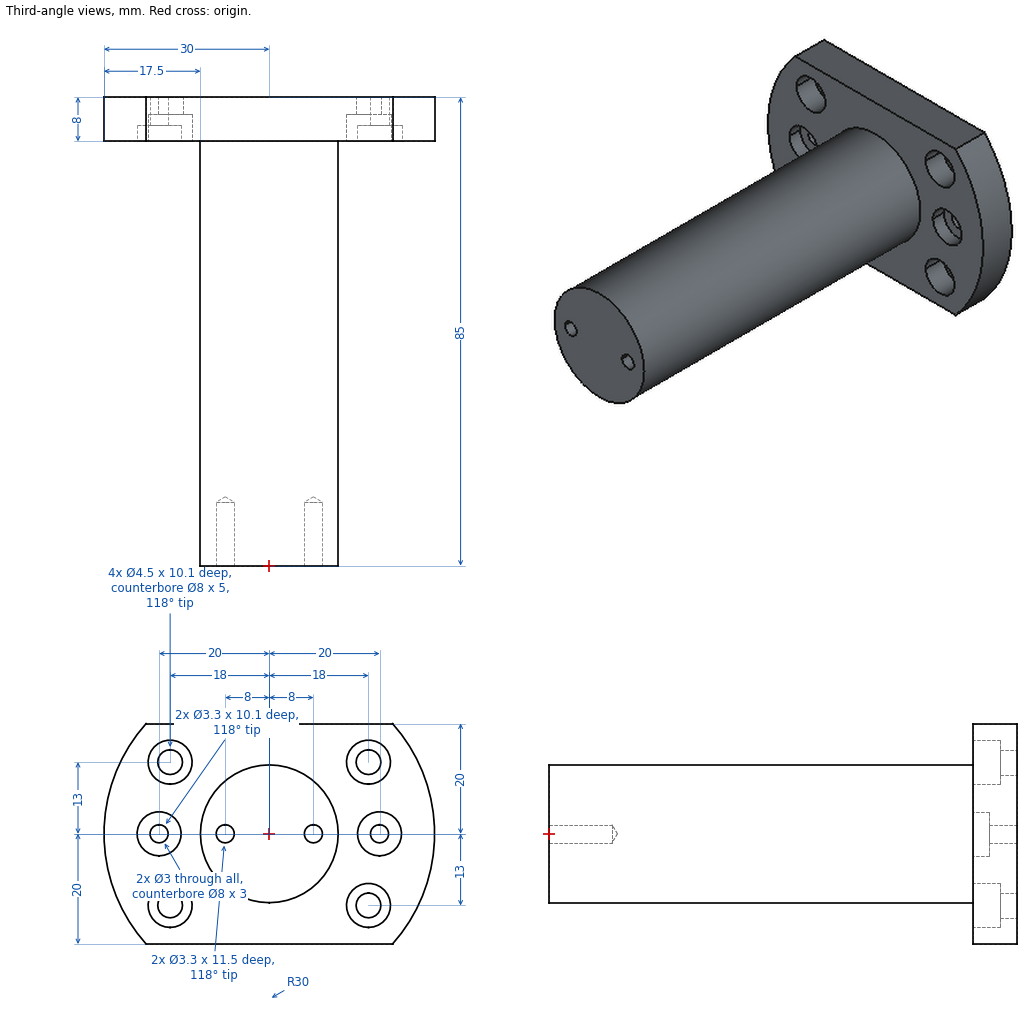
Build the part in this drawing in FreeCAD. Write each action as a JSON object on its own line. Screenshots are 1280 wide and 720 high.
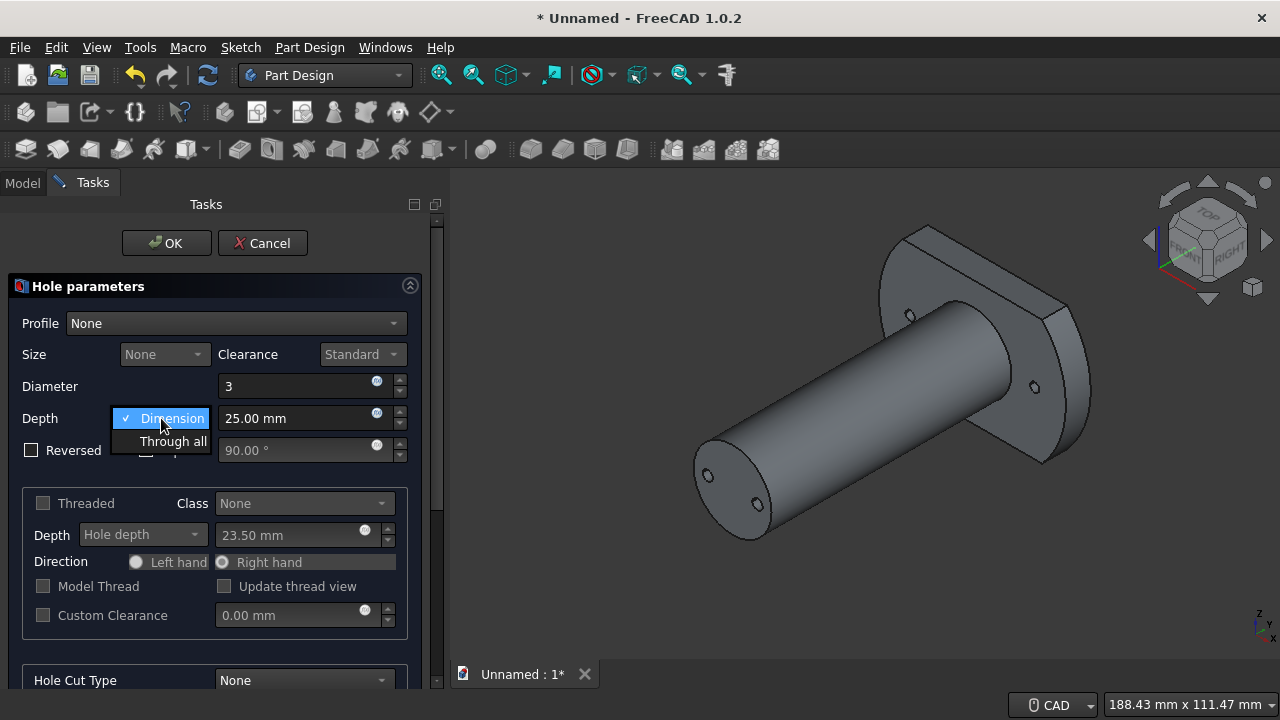
{"action": "left_click", "coordinate": [160, 442]}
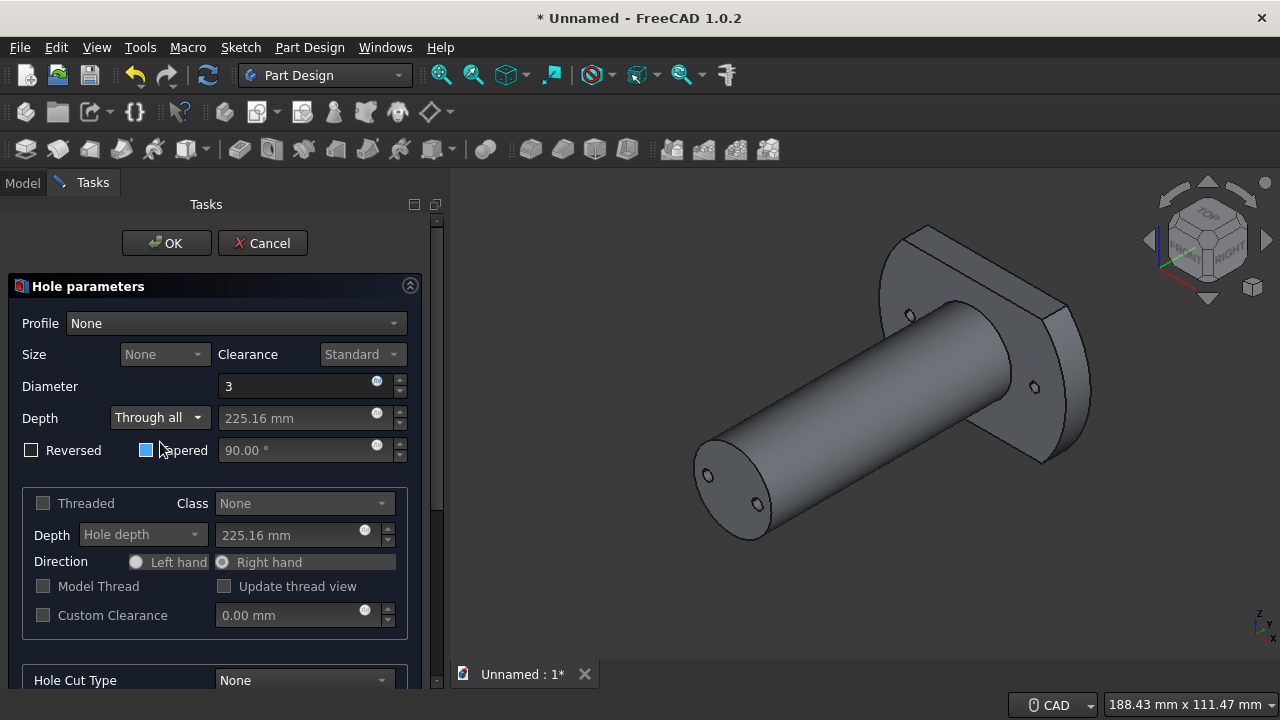
{"action": "scroll", "coordinate": [437, 451], "scroll_direction": "down", "scroll_amount": 2}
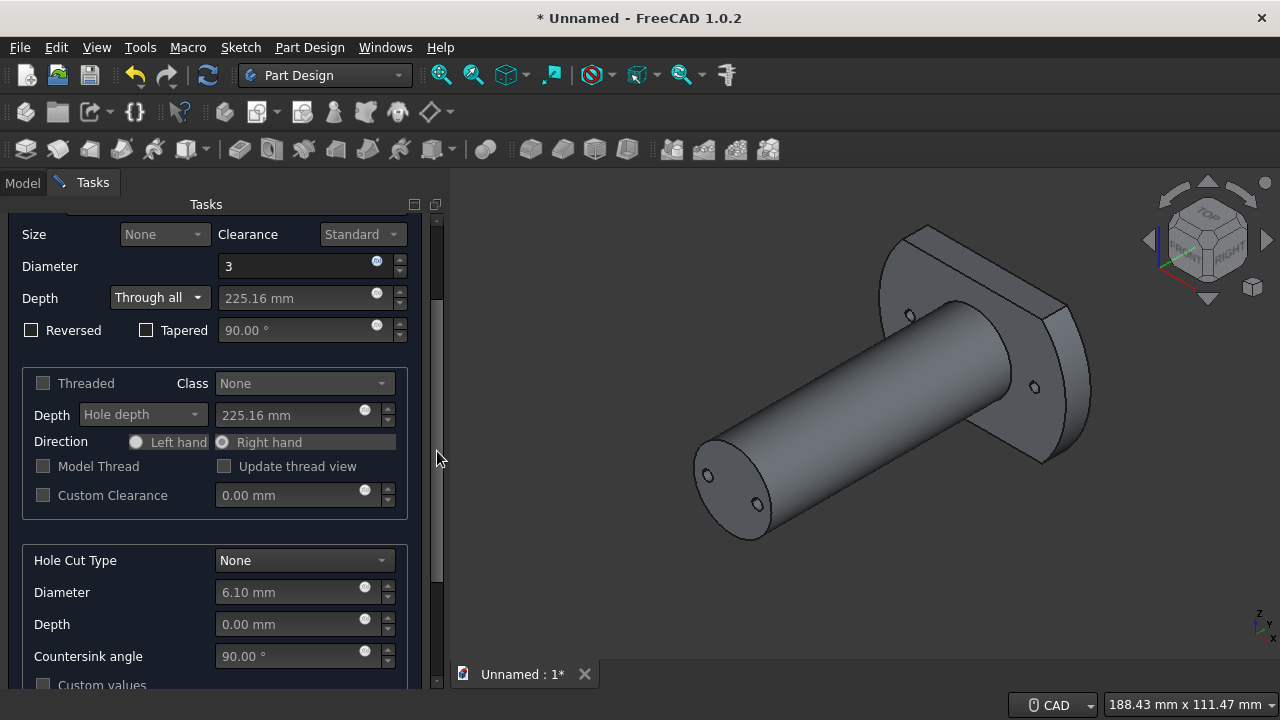
{"action": "left_click", "coordinate": [306, 560]}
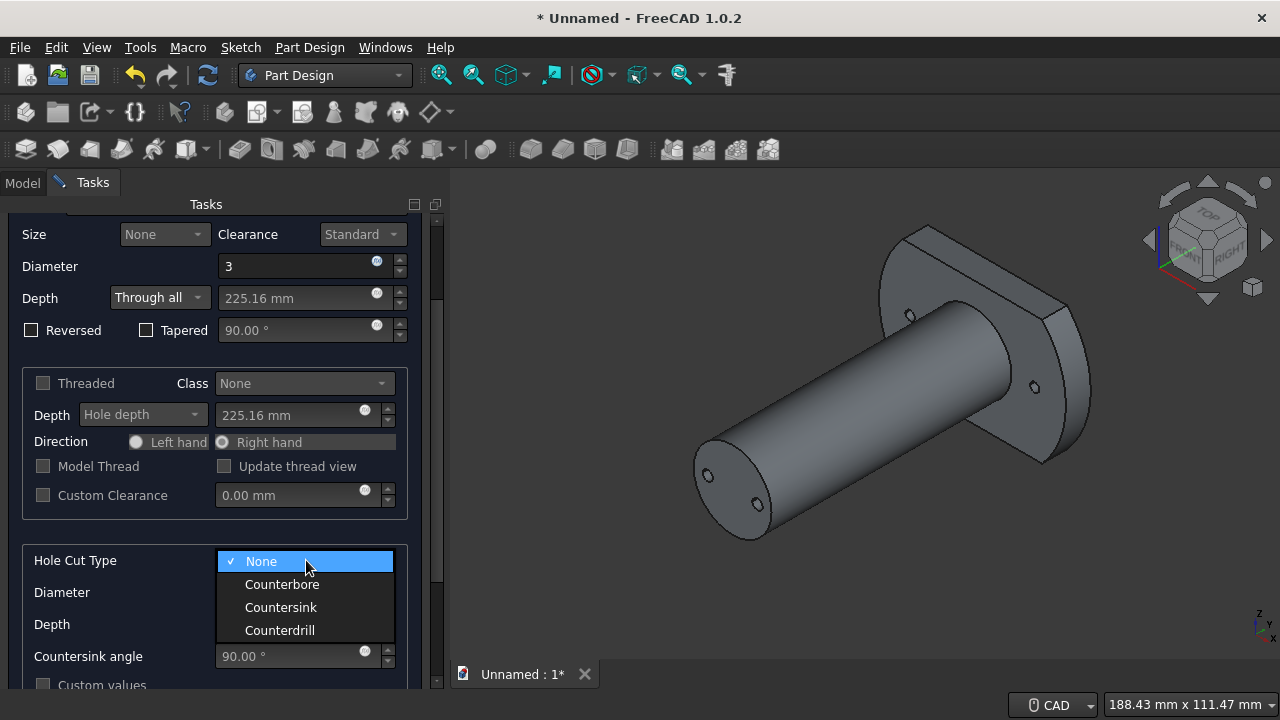
{"action": "left_click", "coordinate": [304, 584]}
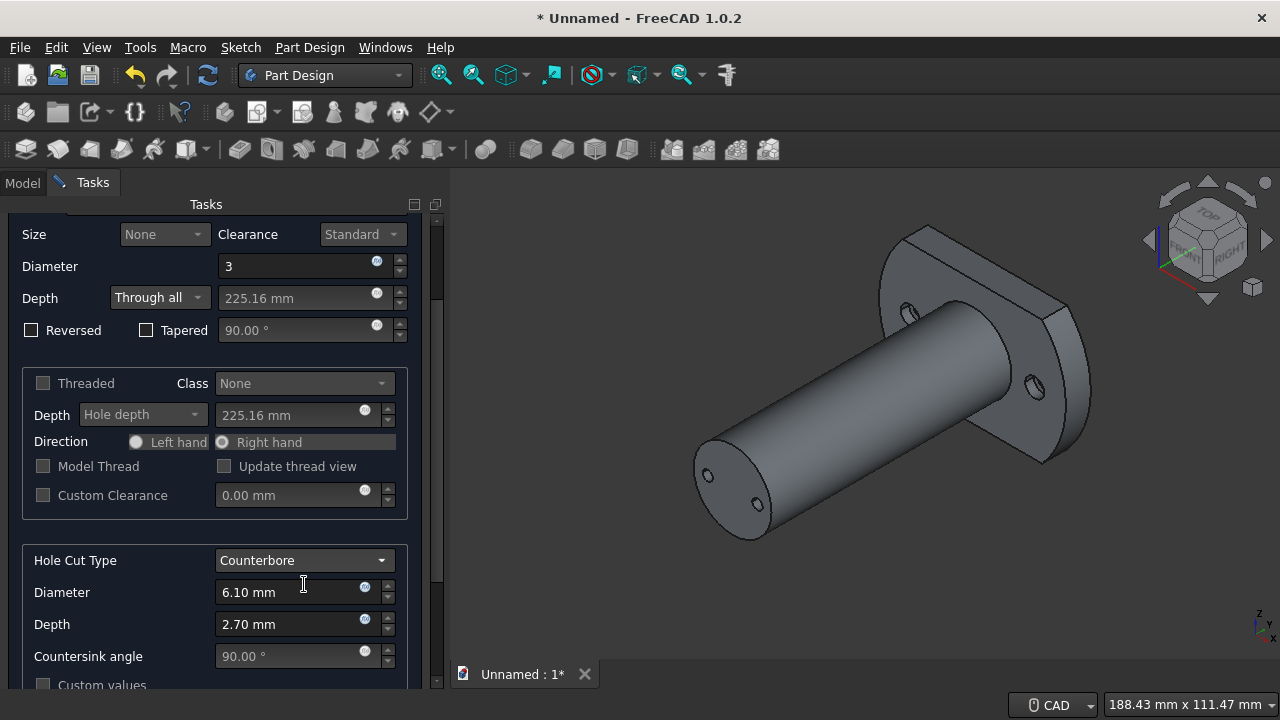
{"action": "triple_click", "coordinate": [298, 592]}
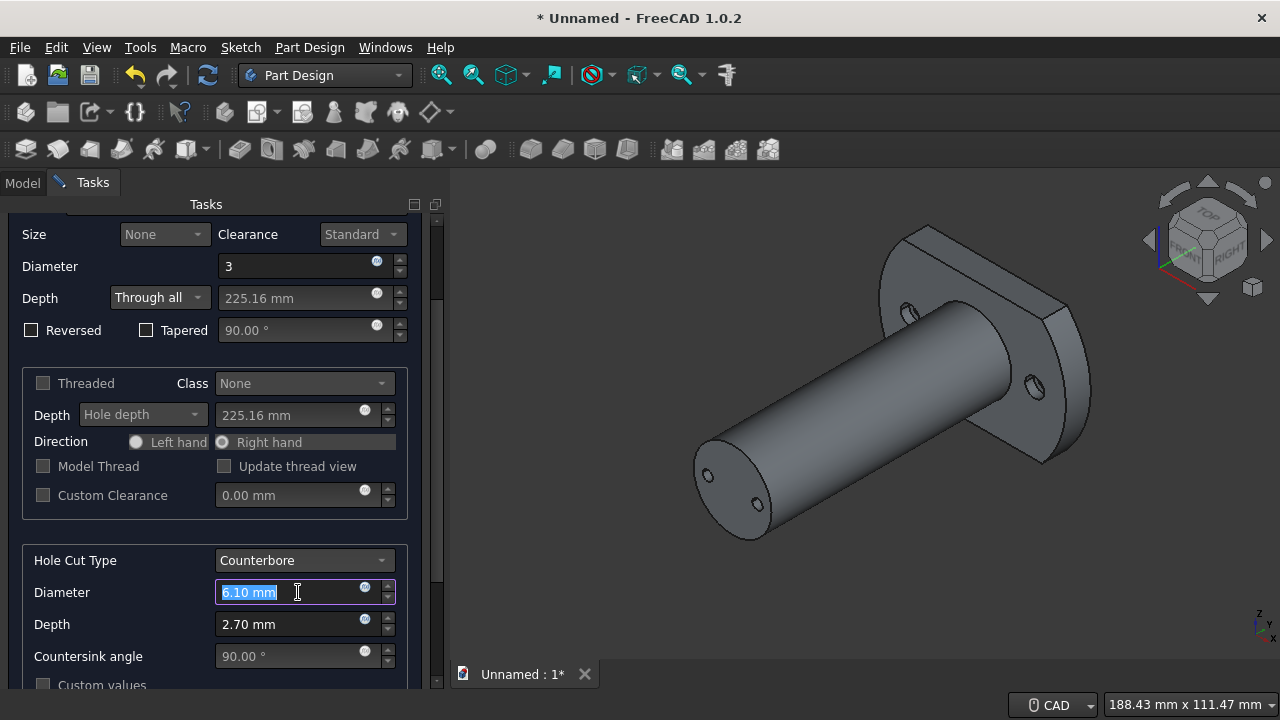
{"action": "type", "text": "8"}
{"action": "key", "text": "Tab"}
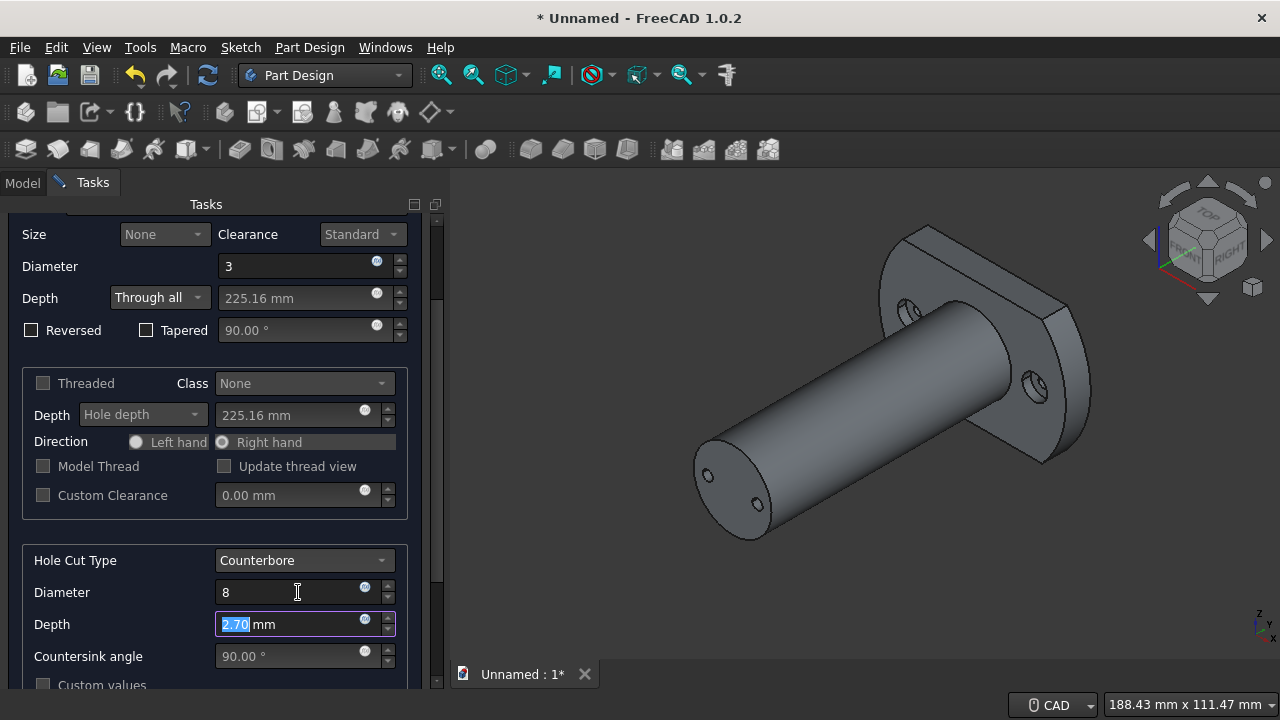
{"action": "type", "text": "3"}
{"action": "key", "text": "Tab"}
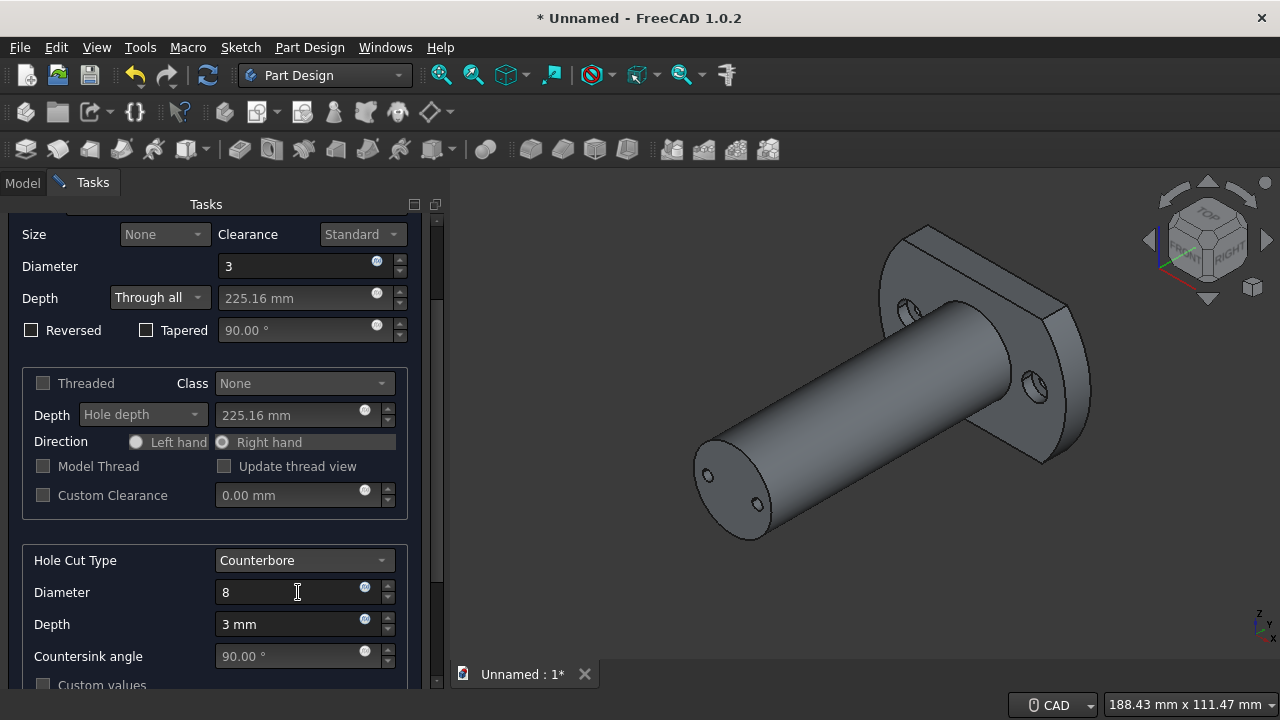
{"action": "scroll", "coordinate": [437, 451], "scroll_direction": "up", "scroll_amount": 3}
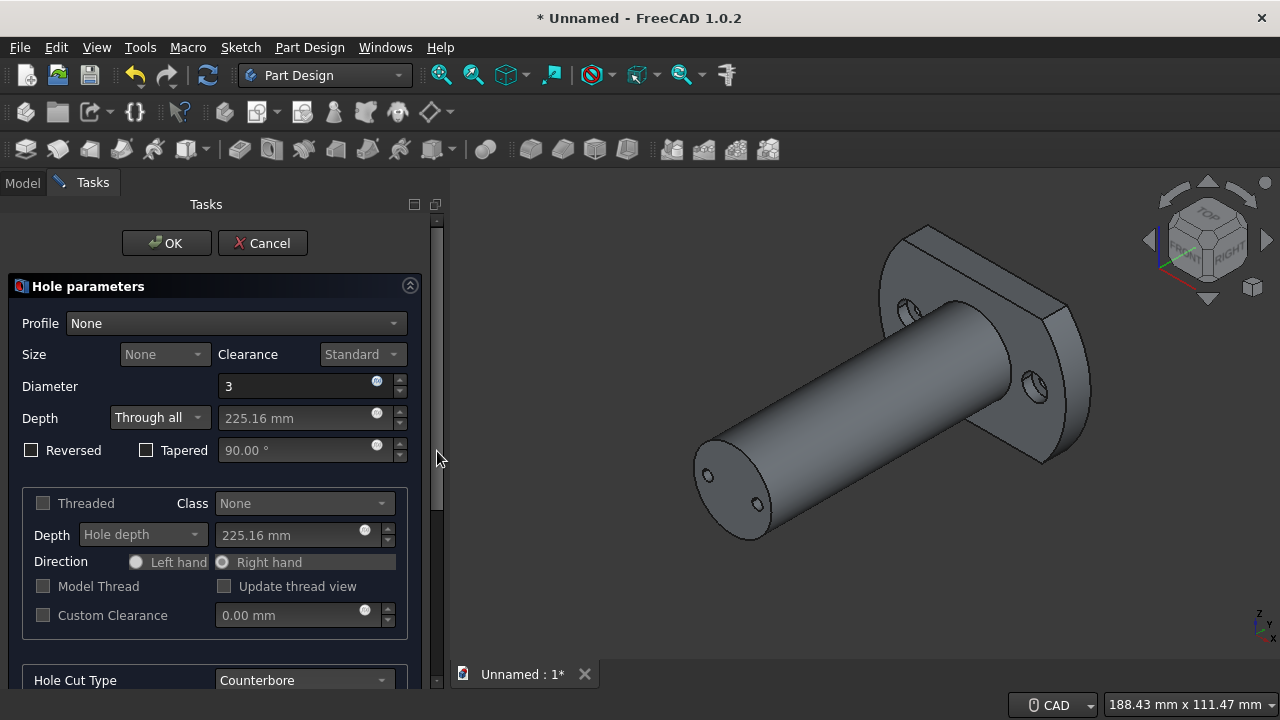
{"action": "left_click", "coordinate": [167, 243]}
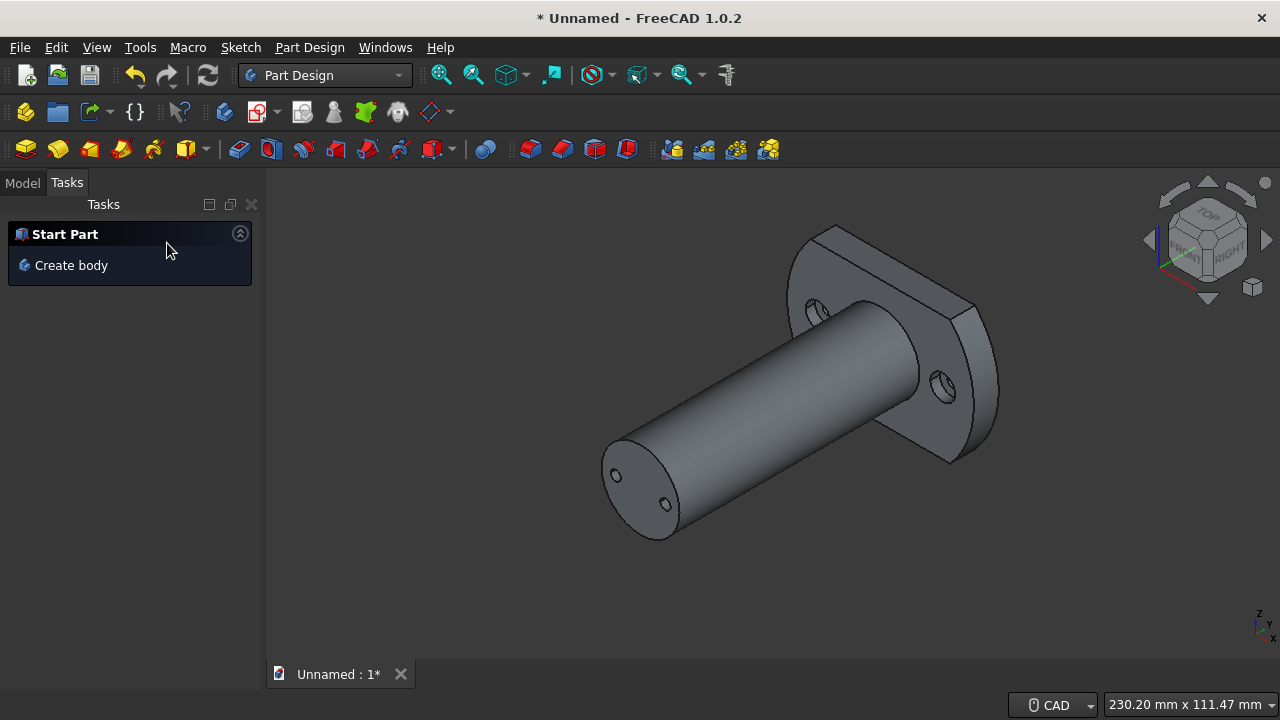
{"action": "scroll", "coordinate": [835, 309], "scroll_direction": "up", "scroll_amount": 5}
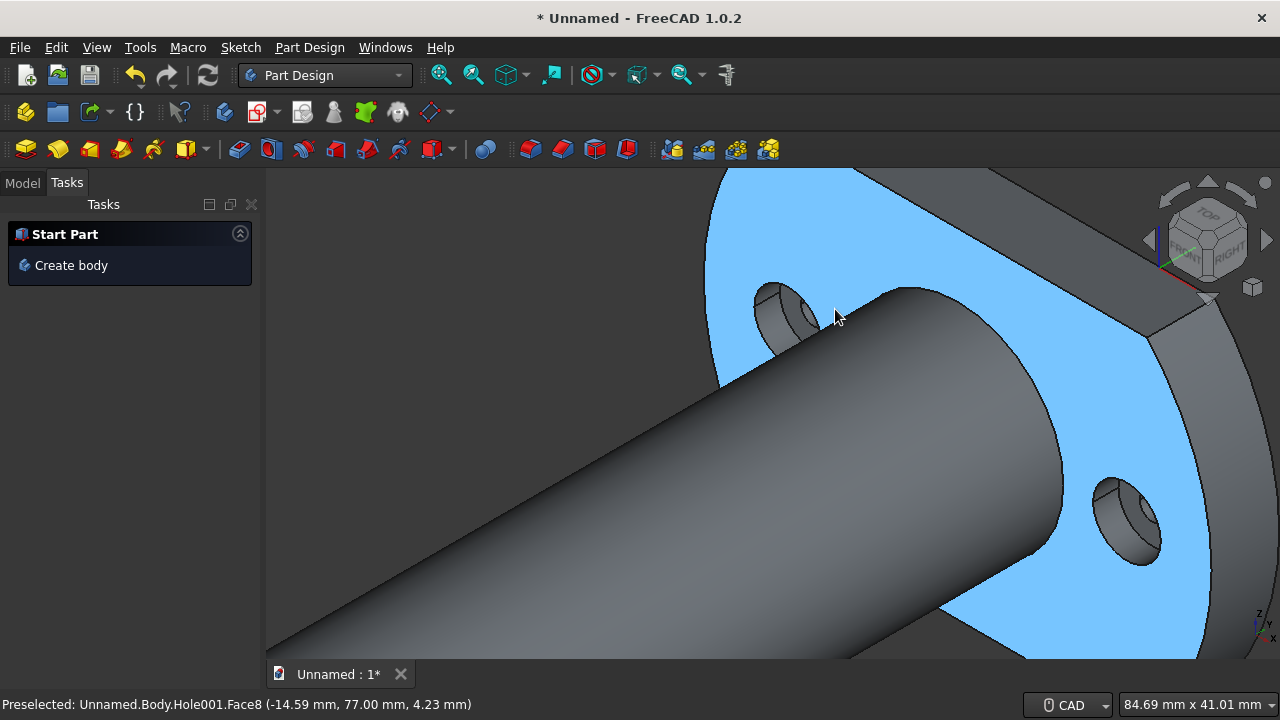
{"action": "left_click", "coordinate": [442, 76]}